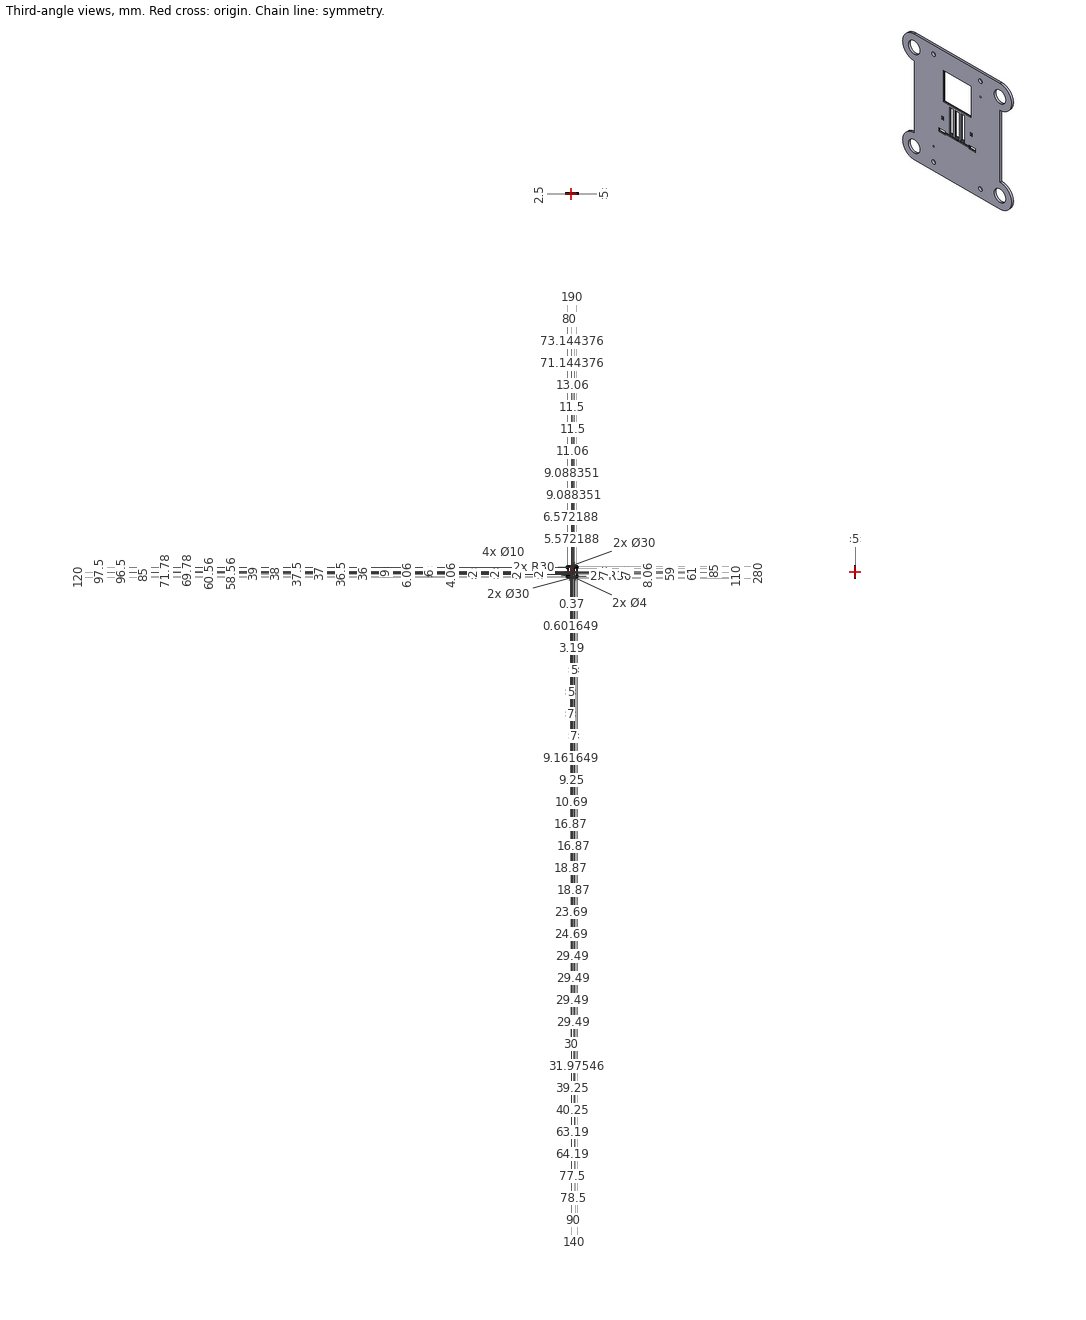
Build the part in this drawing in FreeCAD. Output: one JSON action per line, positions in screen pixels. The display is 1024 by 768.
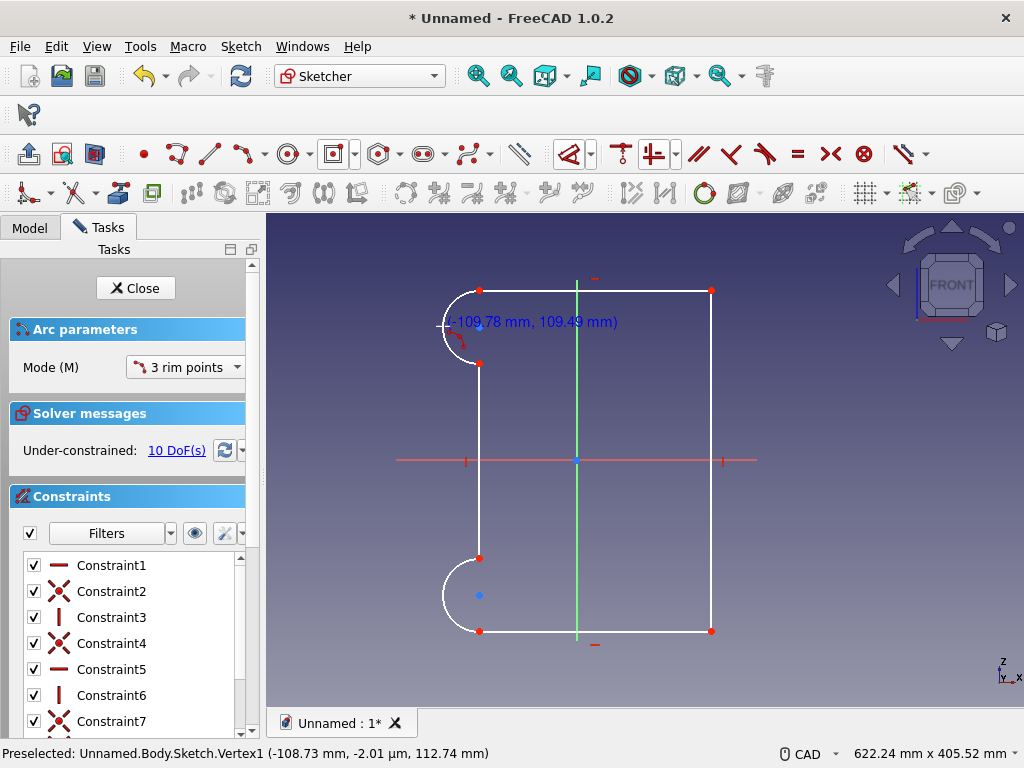
{"action": "left_click", "coordinate": [288, 154]}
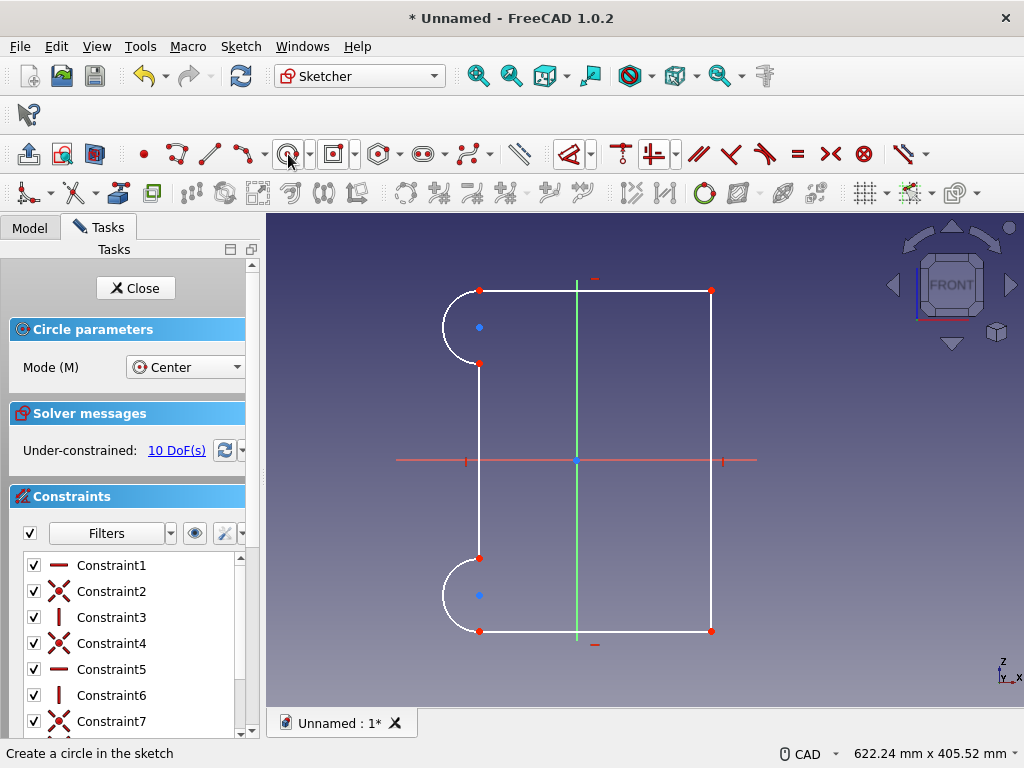
{"action": "scroll", "coordinate": [479, 326], "scroll_direction": "up", "scroll_amount": 2}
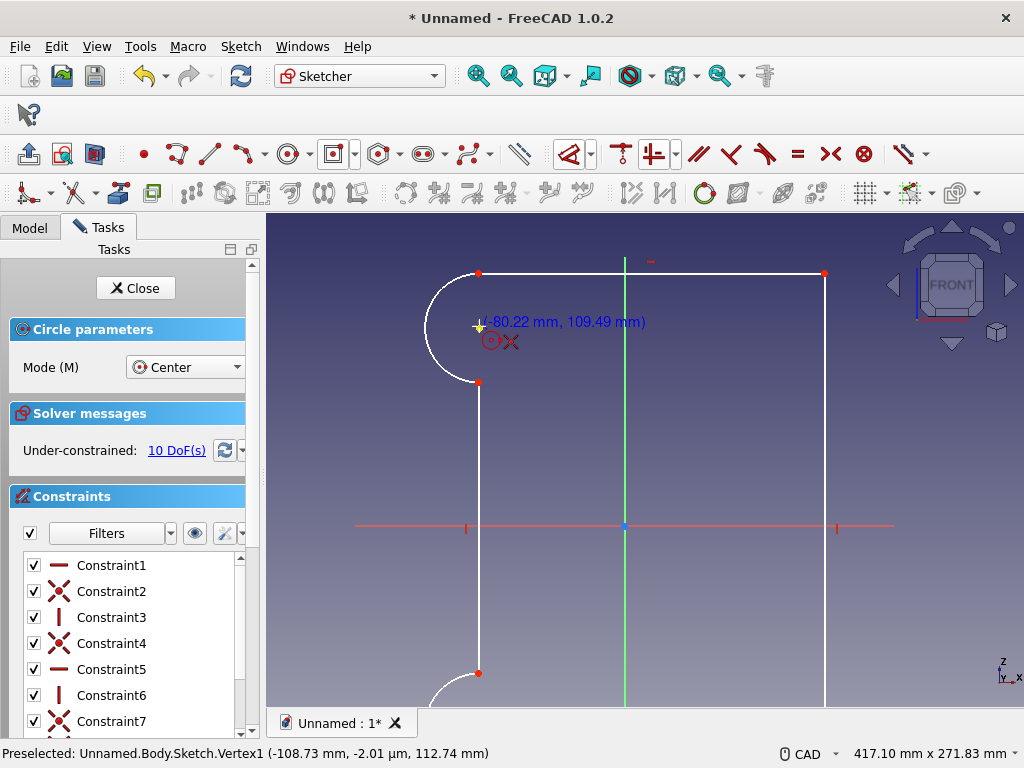
{"action": "left_click", "coordinate": [479, 326]}
{"action": "left_click", "coordinate": [499, 307]}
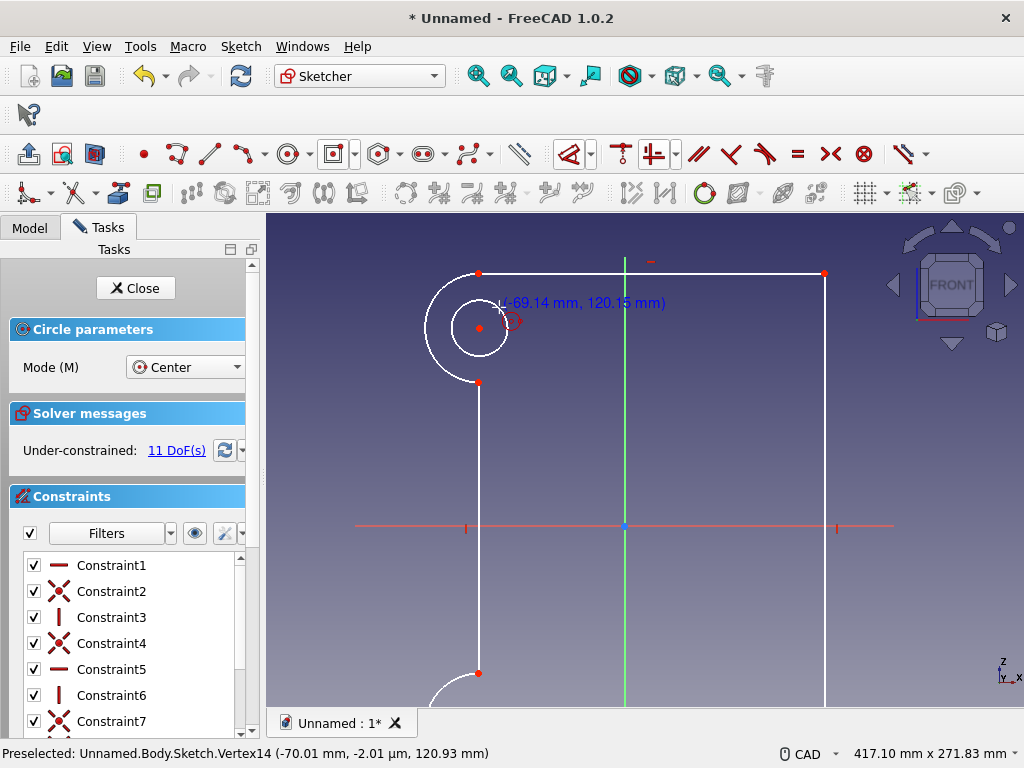
{"action": "scroll", "coordinate": [479, 325], "scroll_direction": "down", "scroll_amount": 2}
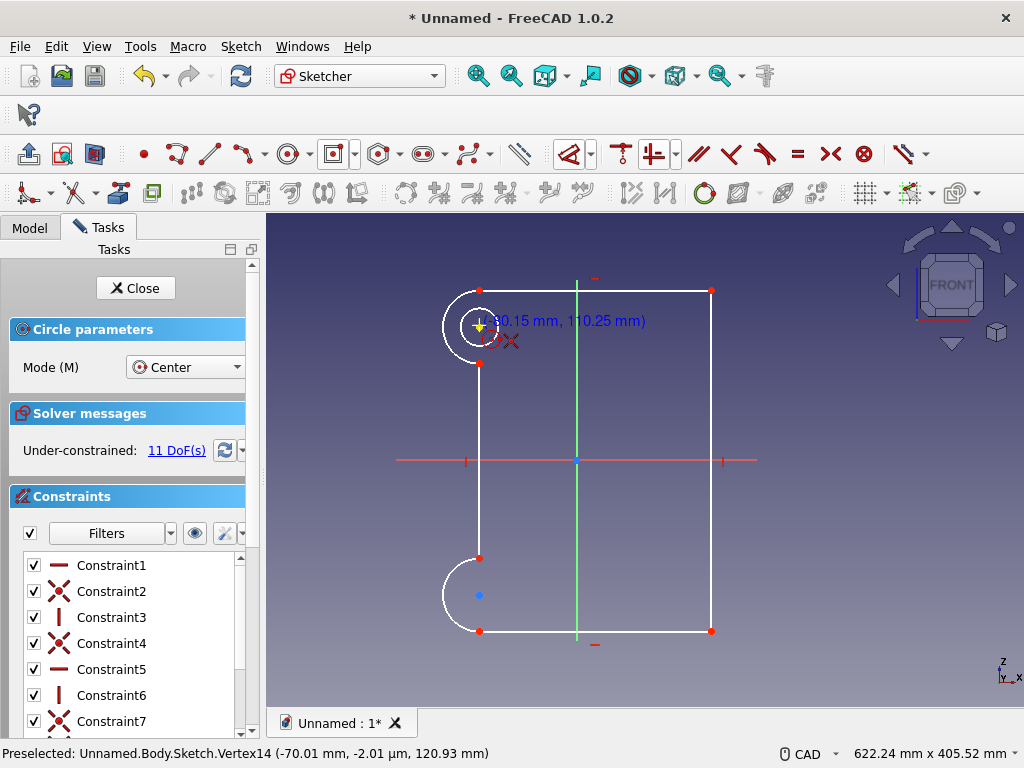
{"action": "scroll", "coordinate": [479, 594], "scroll_direction": "up", "scroll_amount": 2}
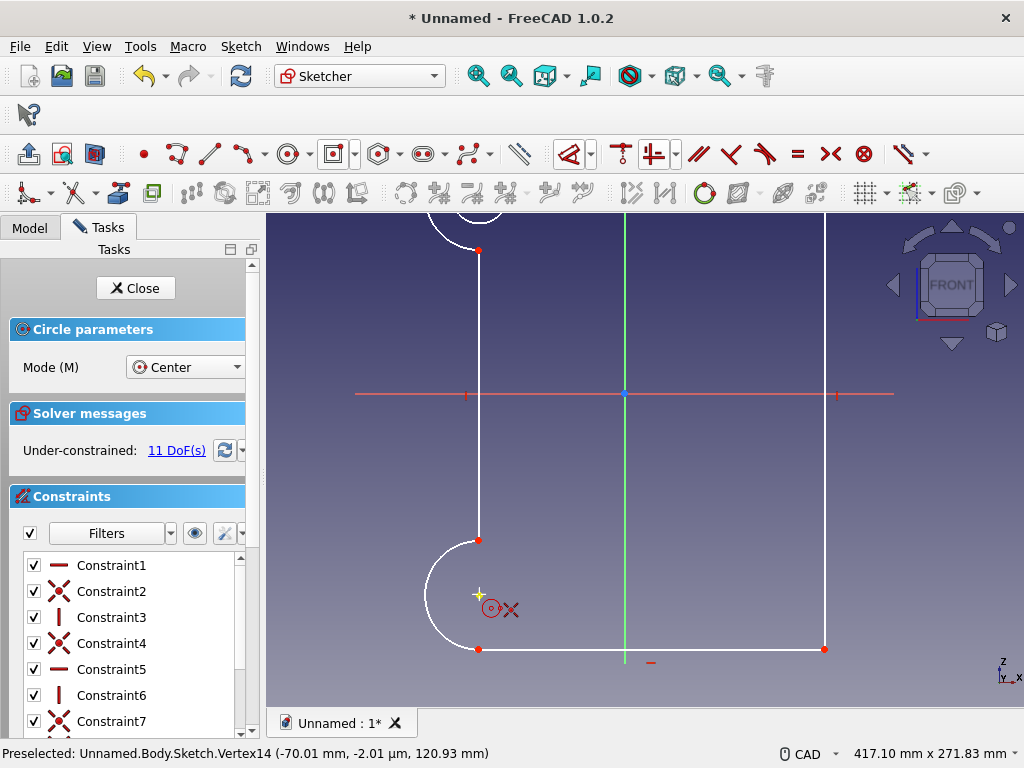
{"action": "left_click", "coordinate": [479, 594]}
{"action": "left_click", "coordinate": [499, 574]}
{"action": "key", "text": "Escape"}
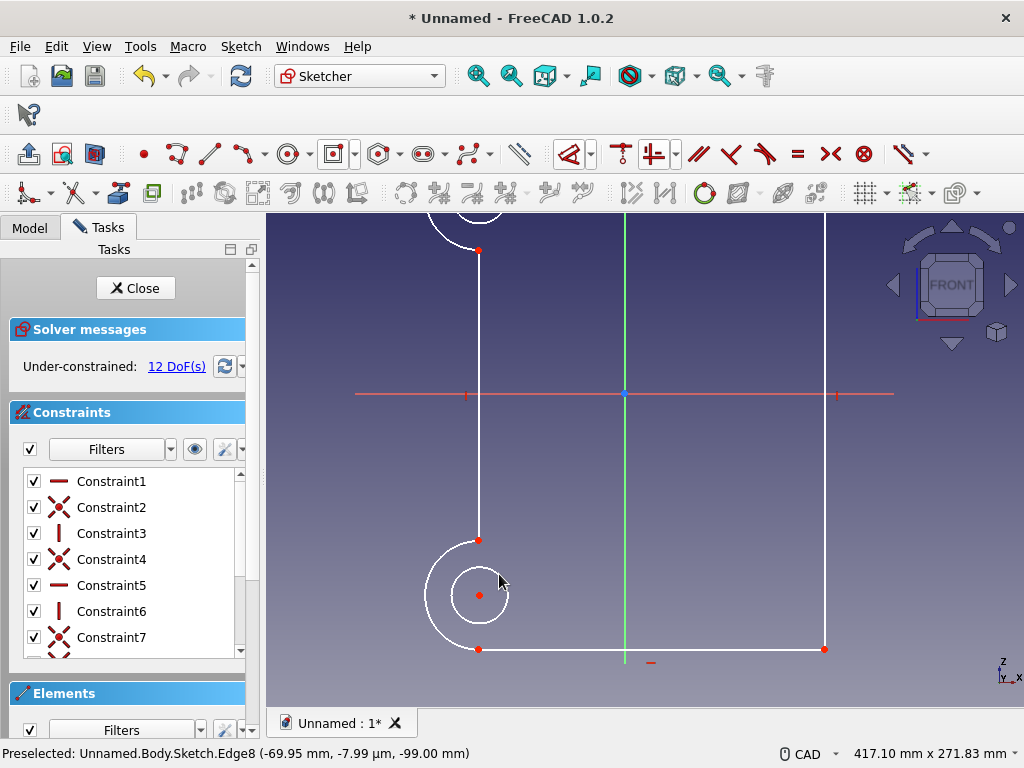
{"action": "scroll", "coordinate": [479, 595], "scroll_direction": "down", "scroll_amount": 2}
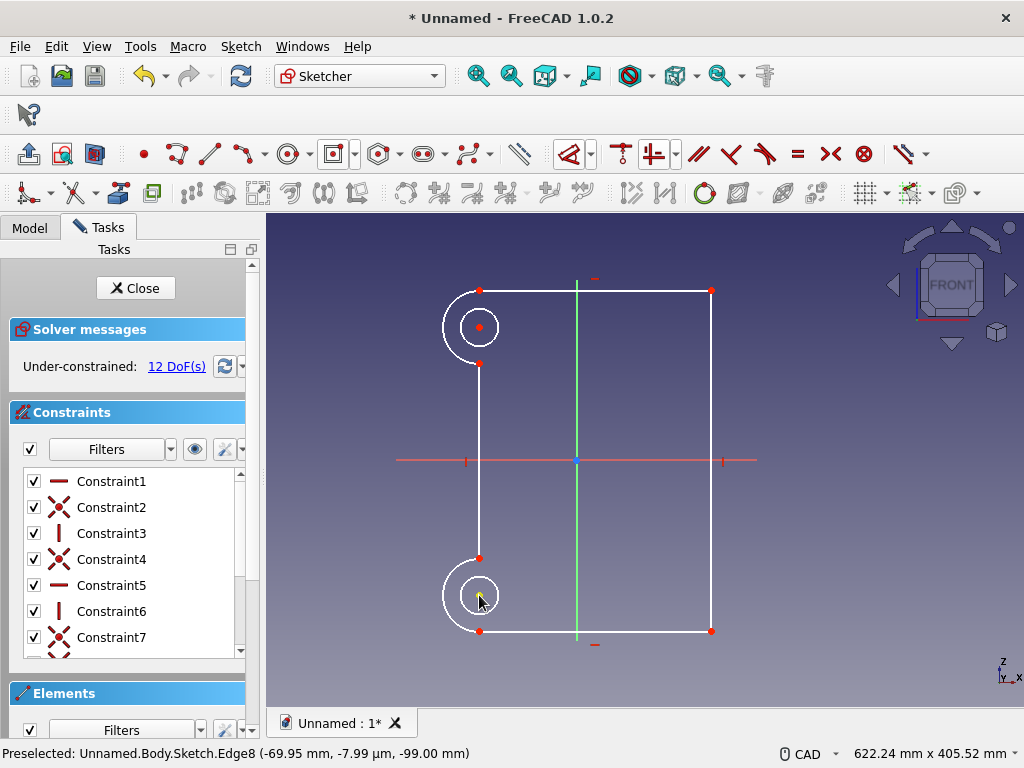
{"action": "left_click", "coordinate": [549, 291]}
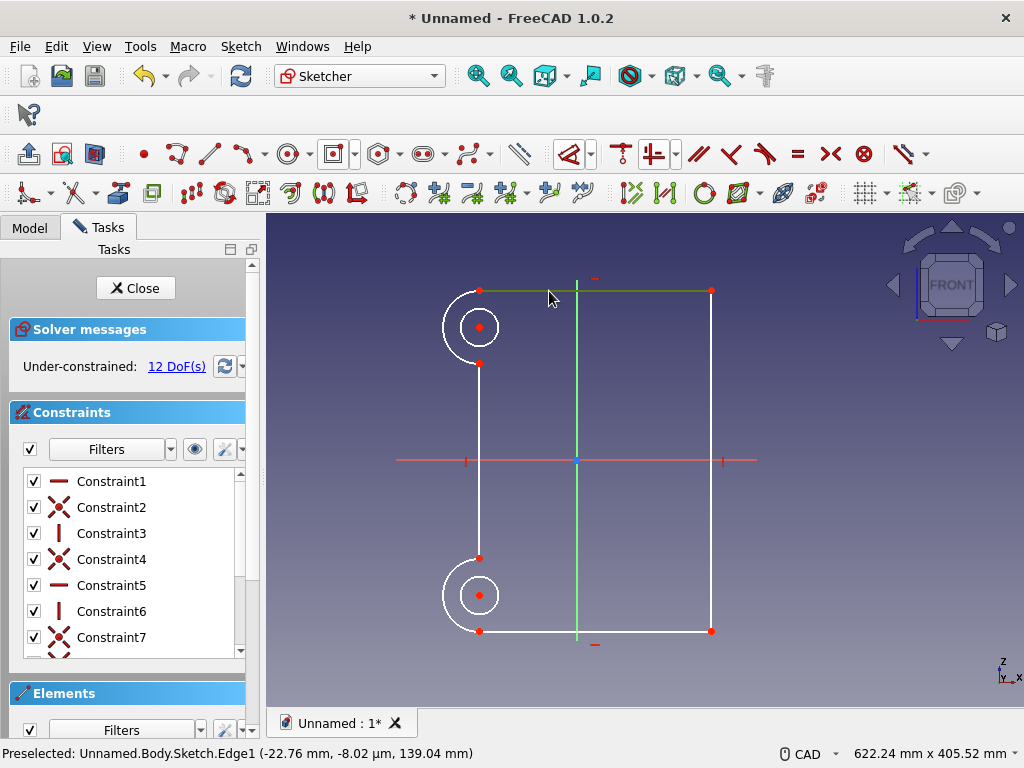
{"action": "left_click", "coordinate": [450, 306]}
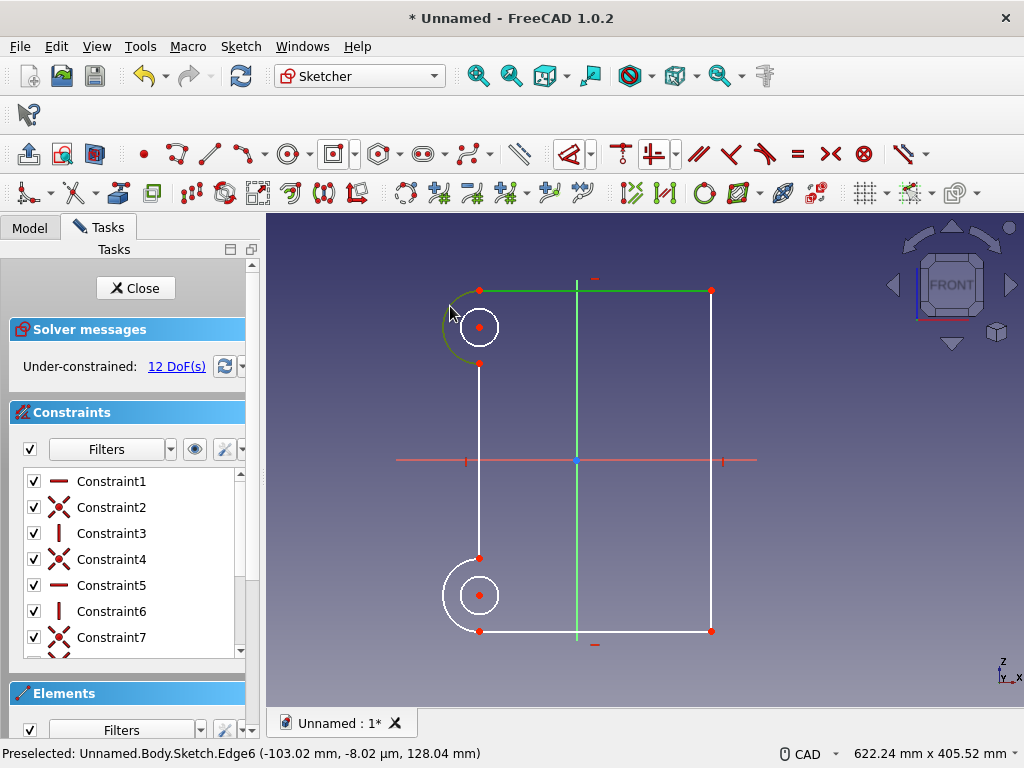
{"action": "left_click", "coordinate": [765, 154]}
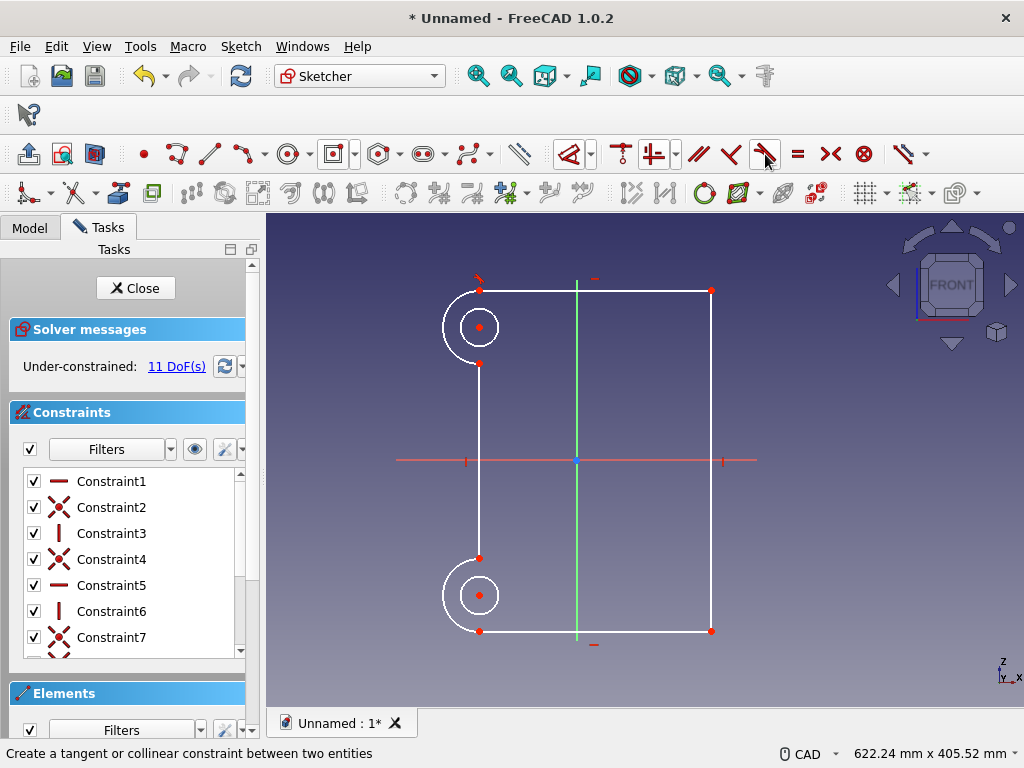
{"action": "left_click", "coordinate": [641, 632]}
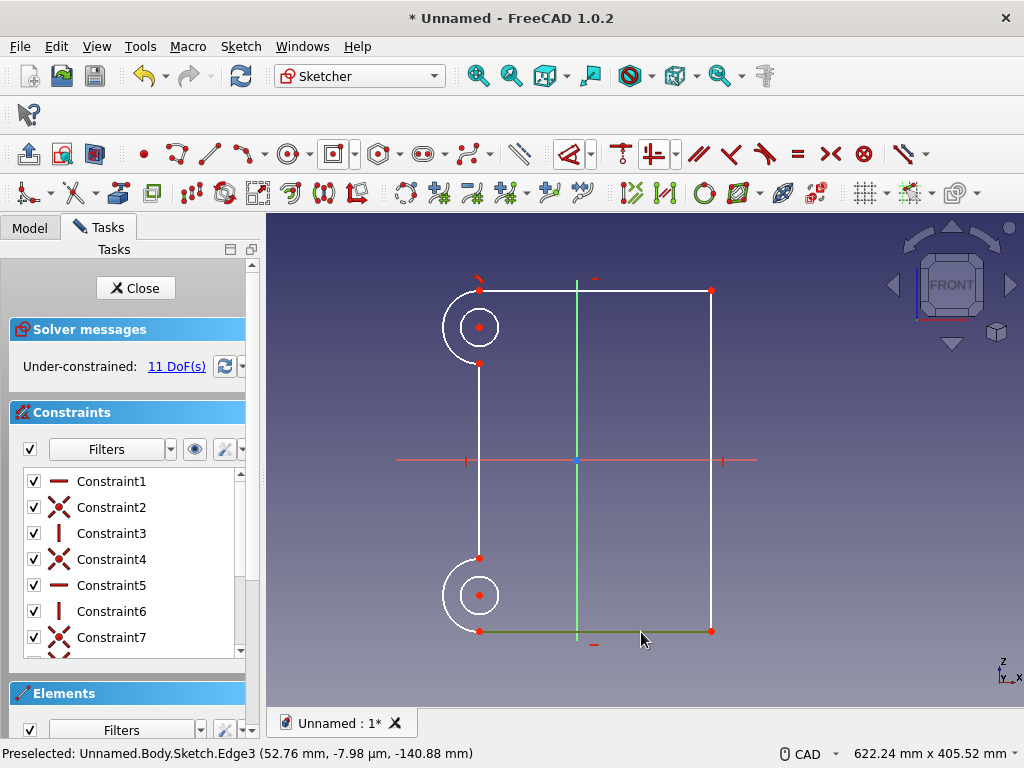
{"action": "left_click", "coordinate": [450, 574]}